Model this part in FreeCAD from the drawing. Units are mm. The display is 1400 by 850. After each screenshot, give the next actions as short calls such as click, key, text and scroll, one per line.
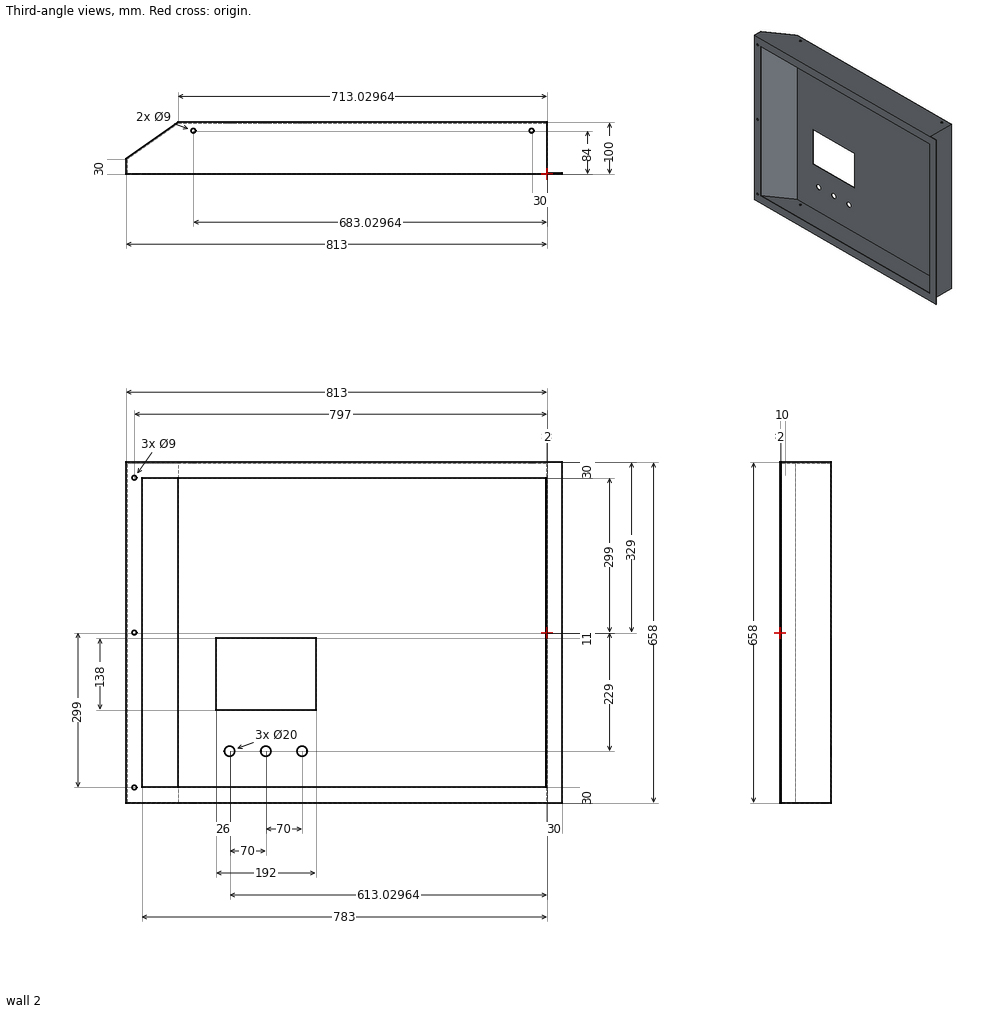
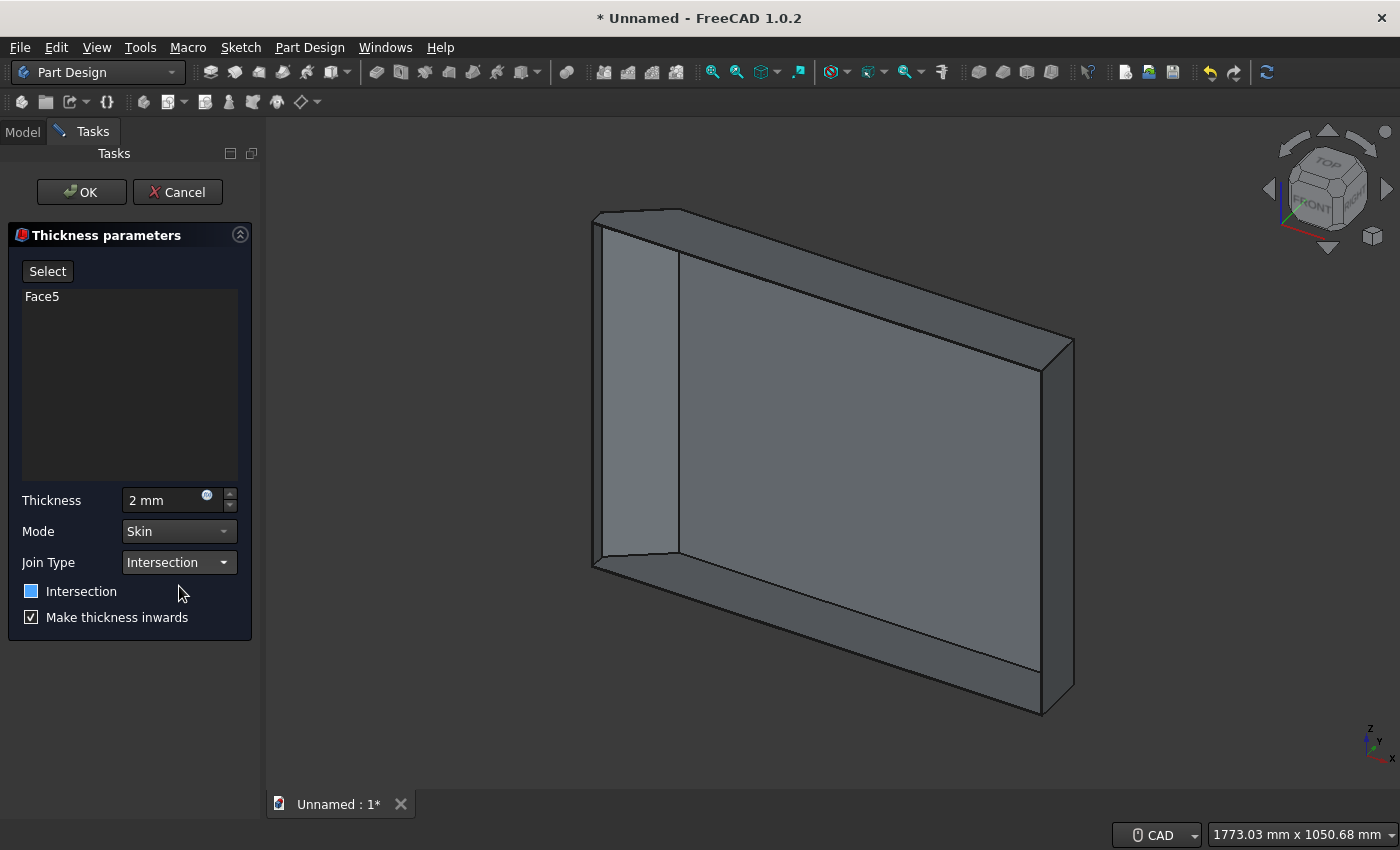
click(82, 192)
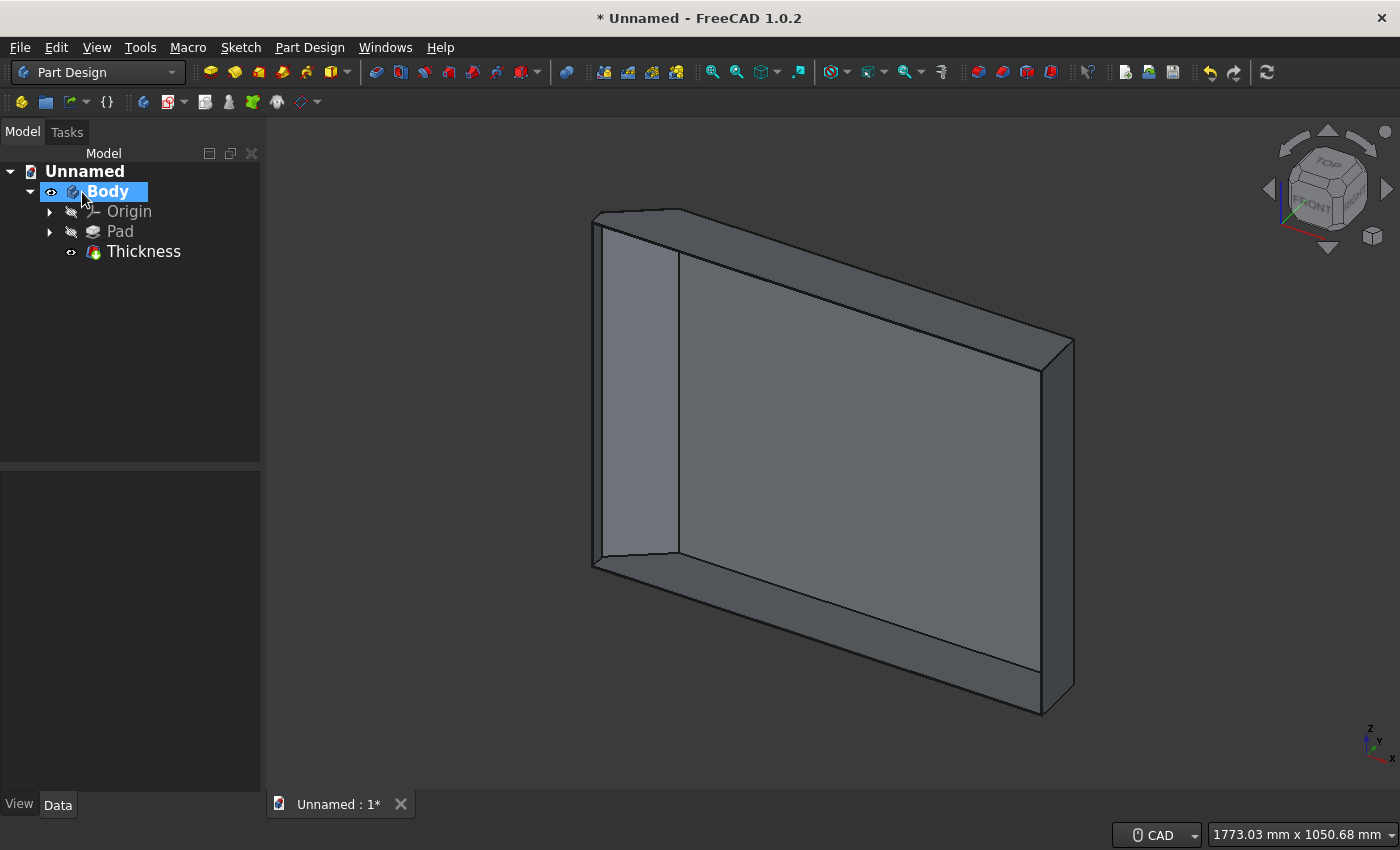
key(4)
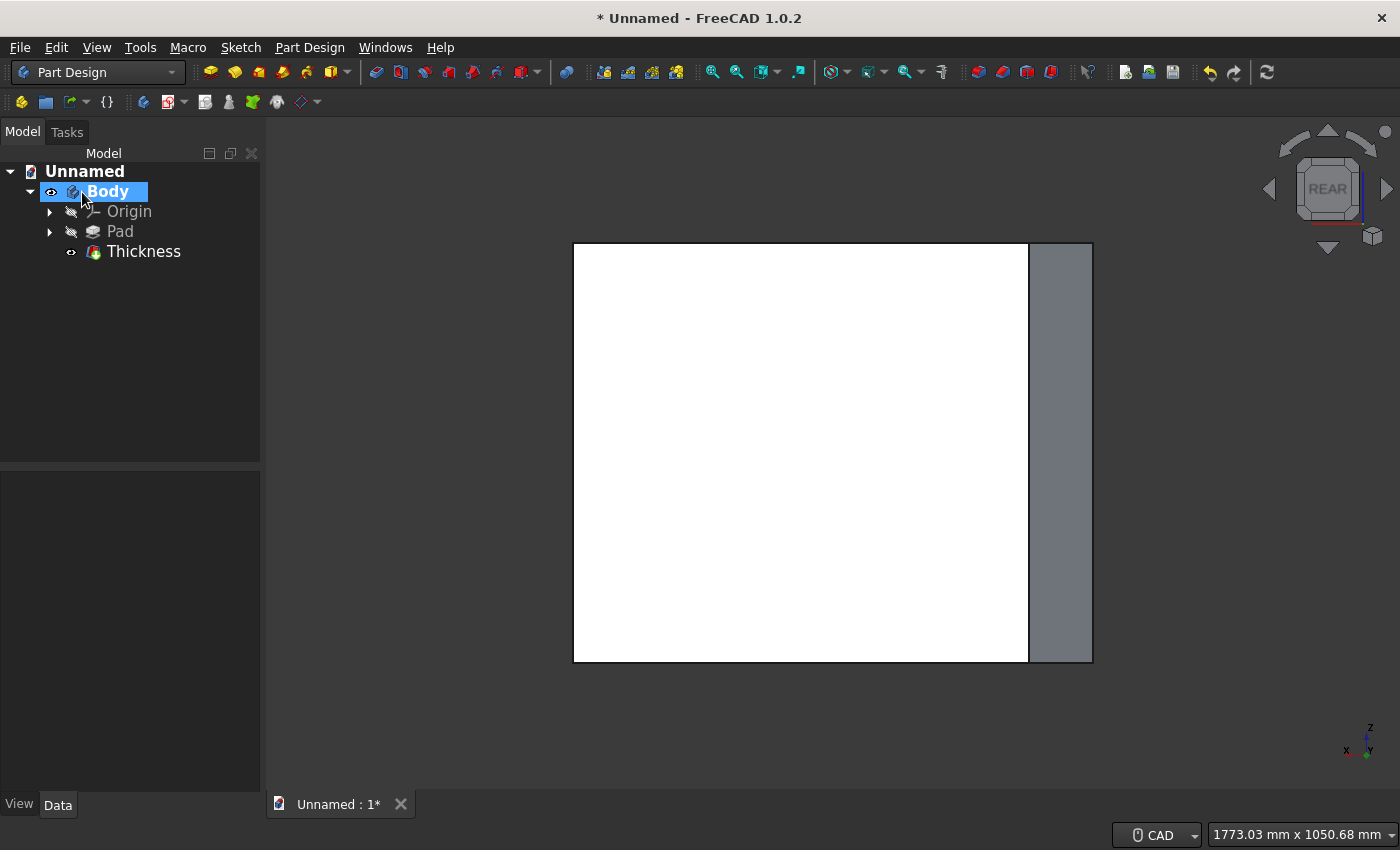
click(801, 452)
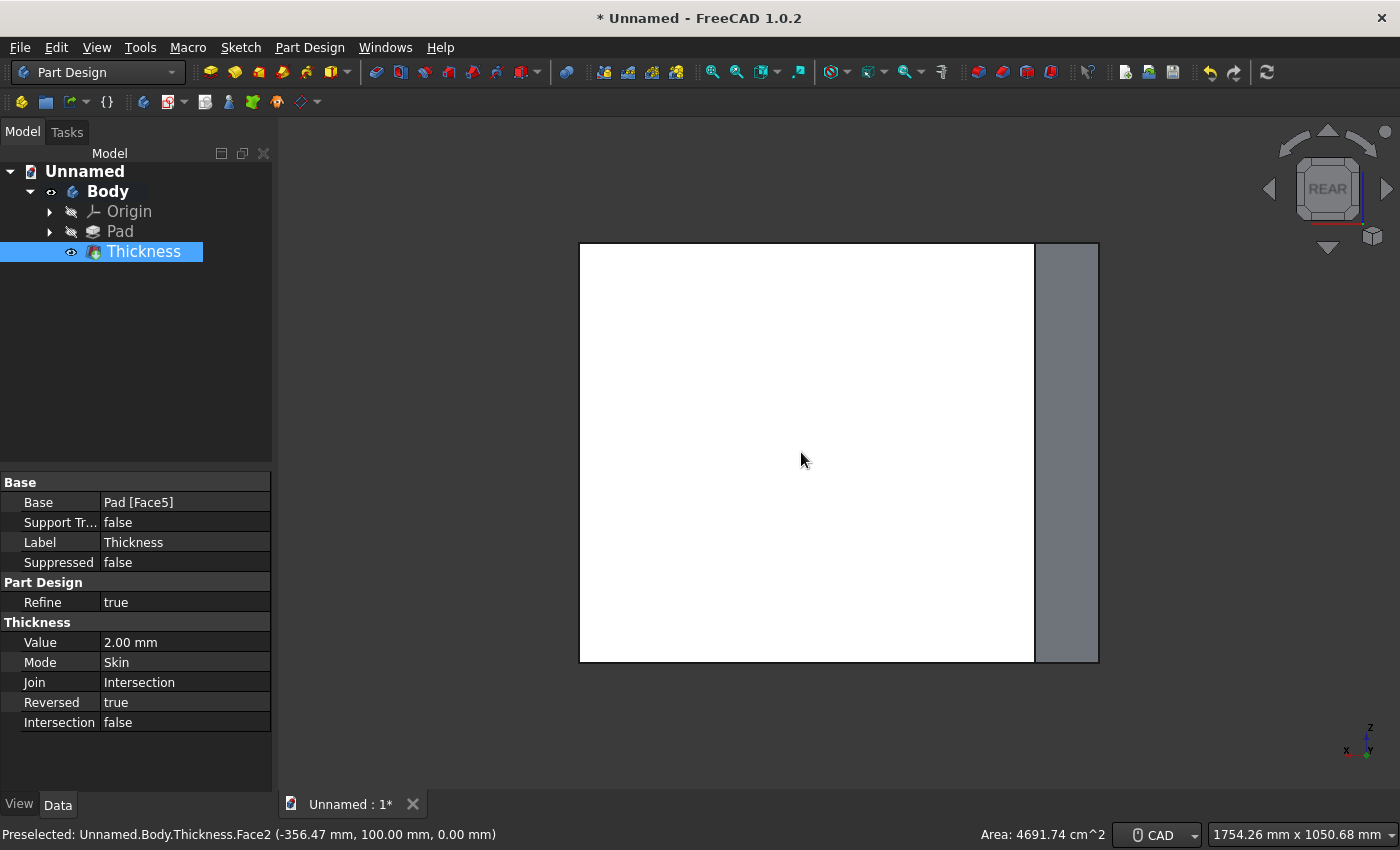
click(168, 102)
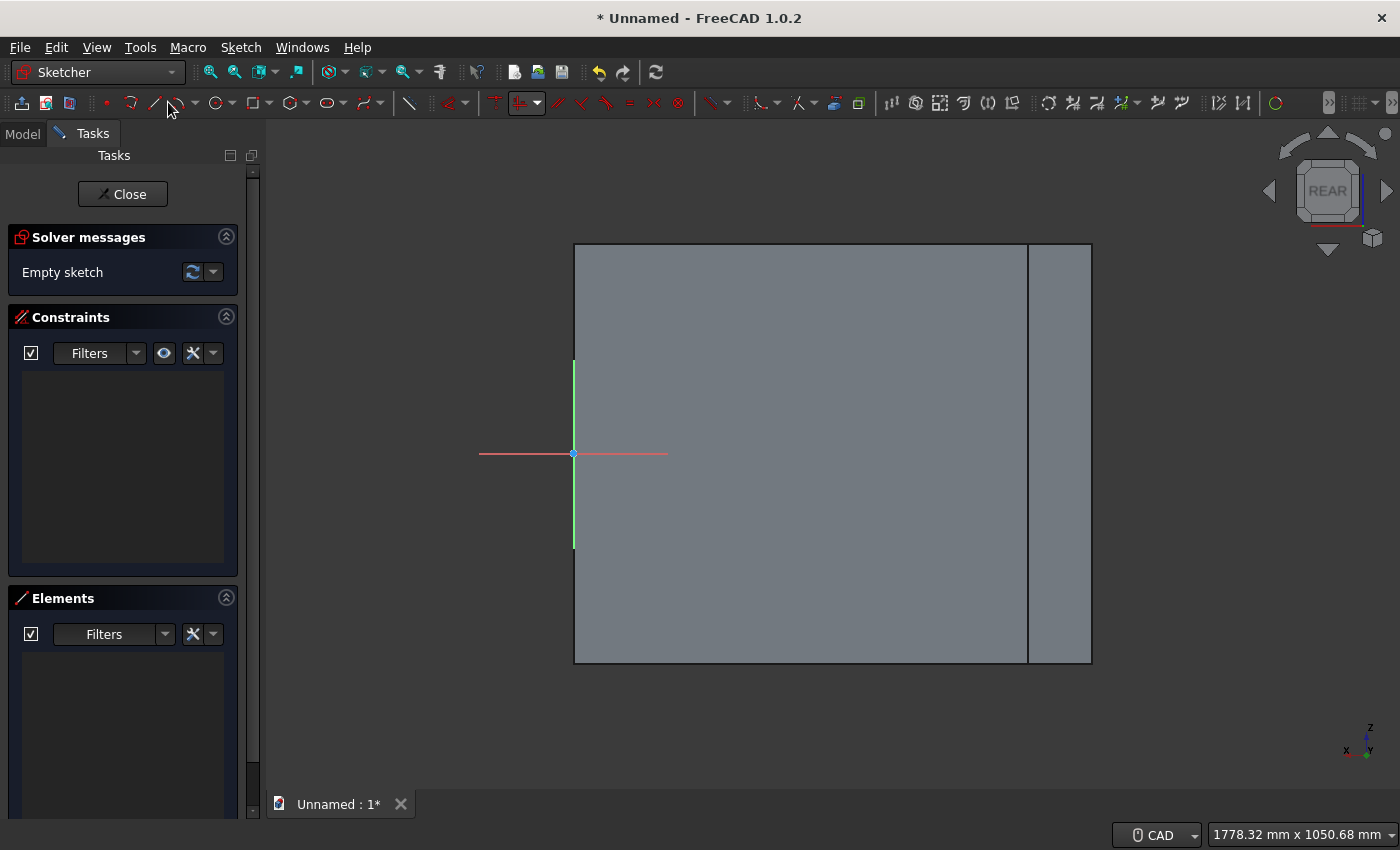
scroll(1011, 580, up, 5)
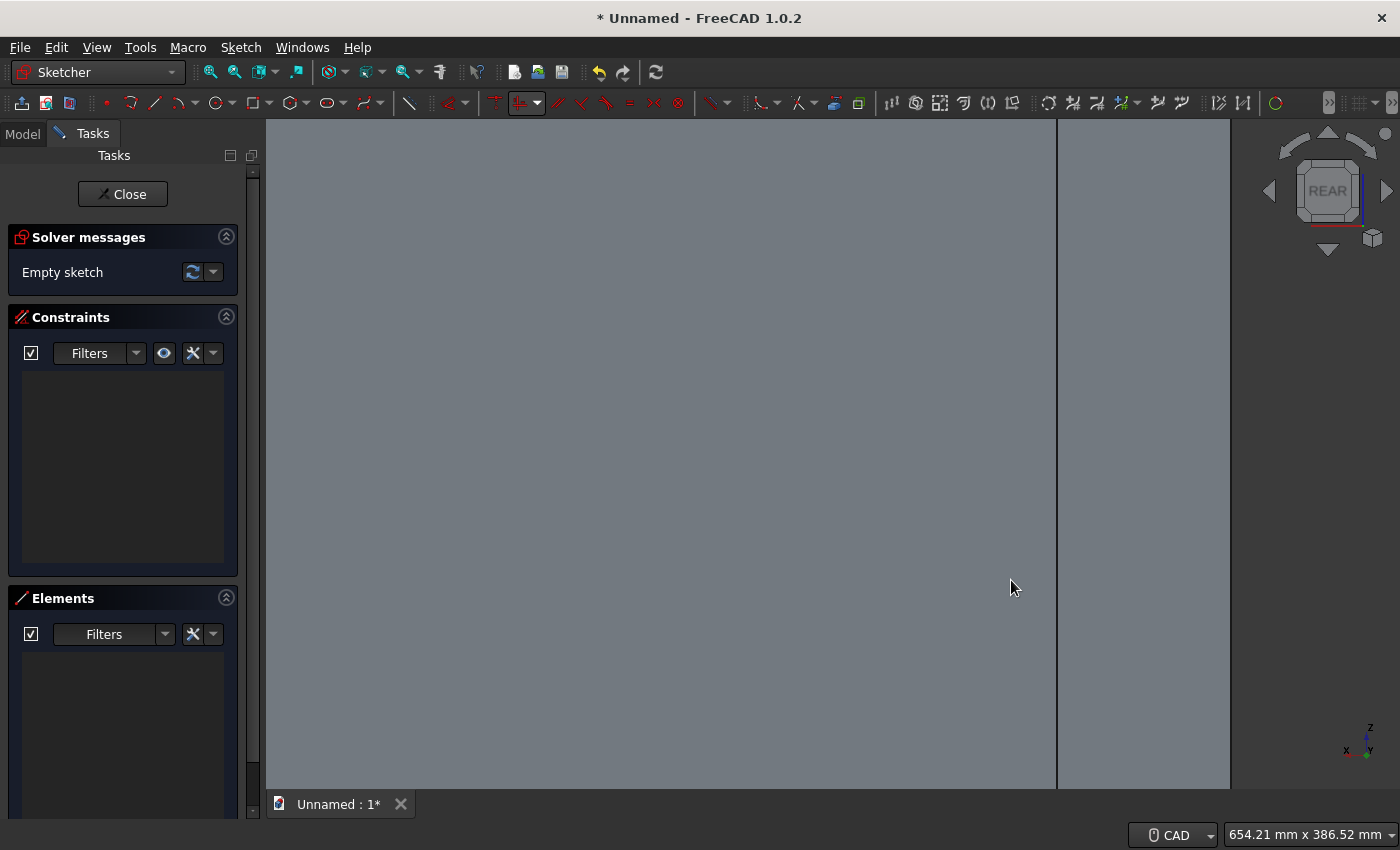
click(254, 104)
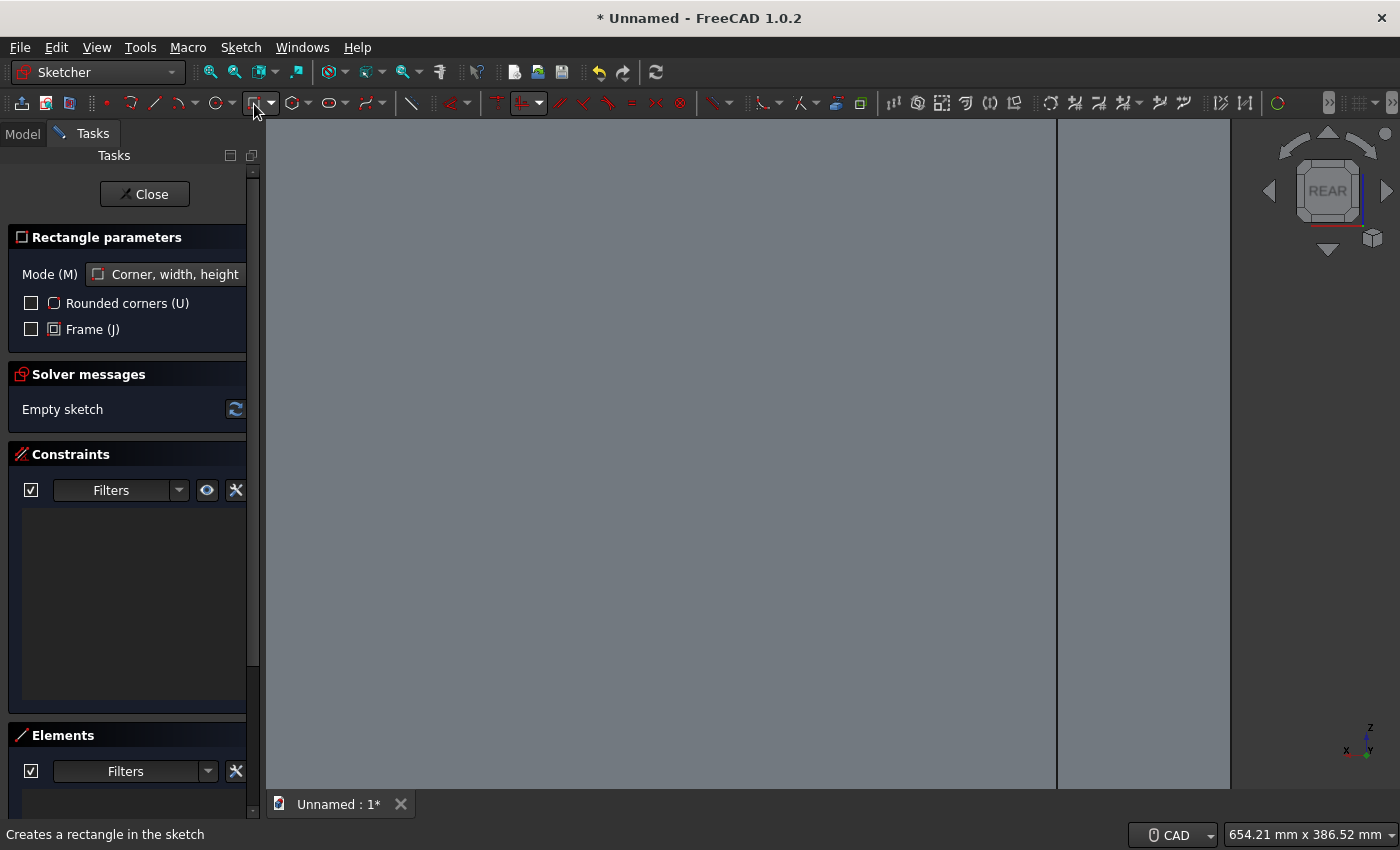
click(596, 255)
click(929, 495)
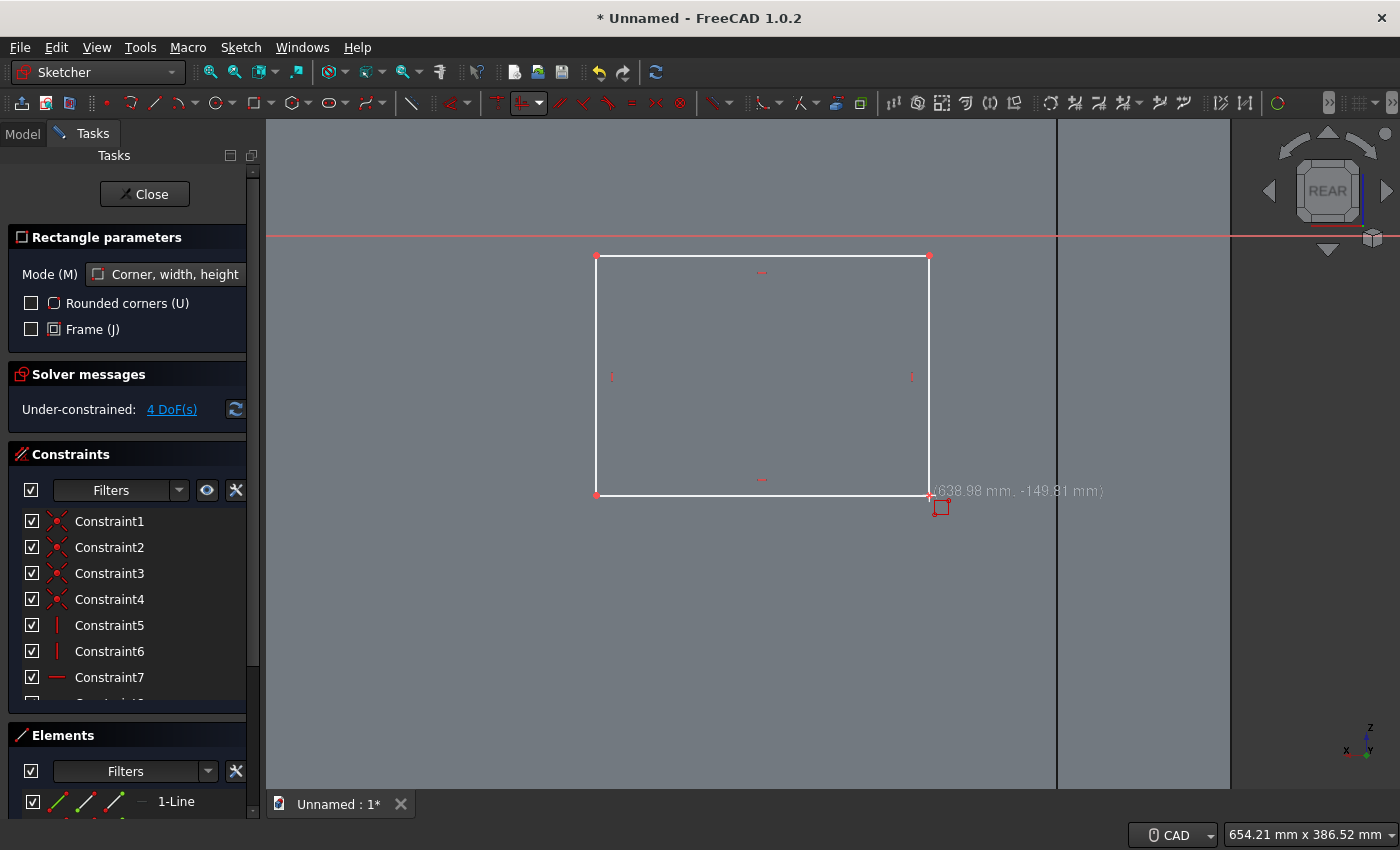
click(216, 104)